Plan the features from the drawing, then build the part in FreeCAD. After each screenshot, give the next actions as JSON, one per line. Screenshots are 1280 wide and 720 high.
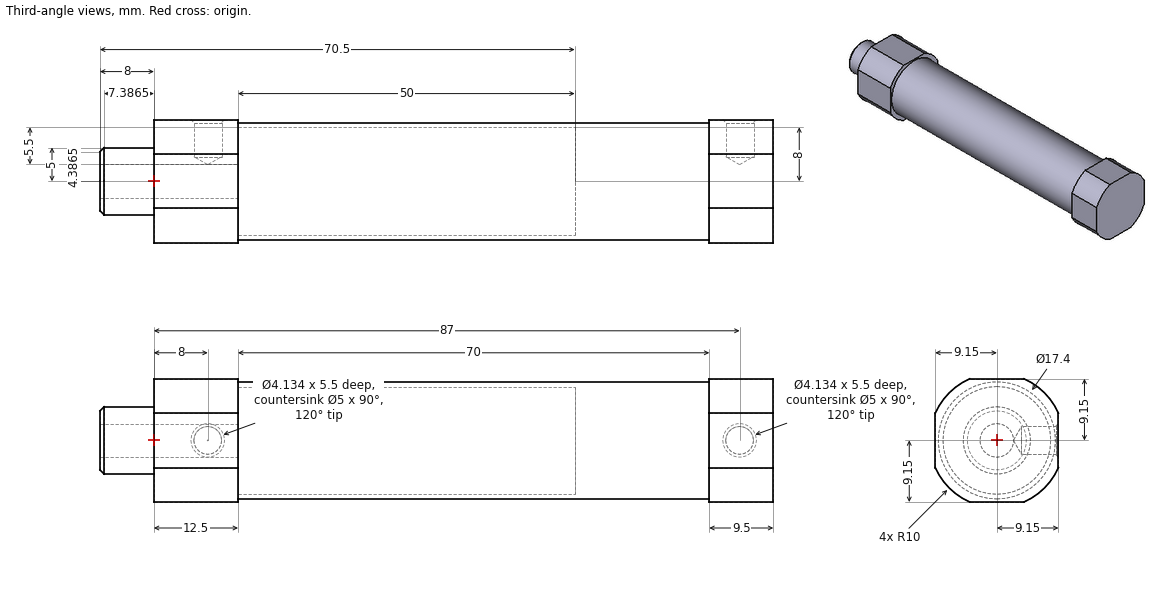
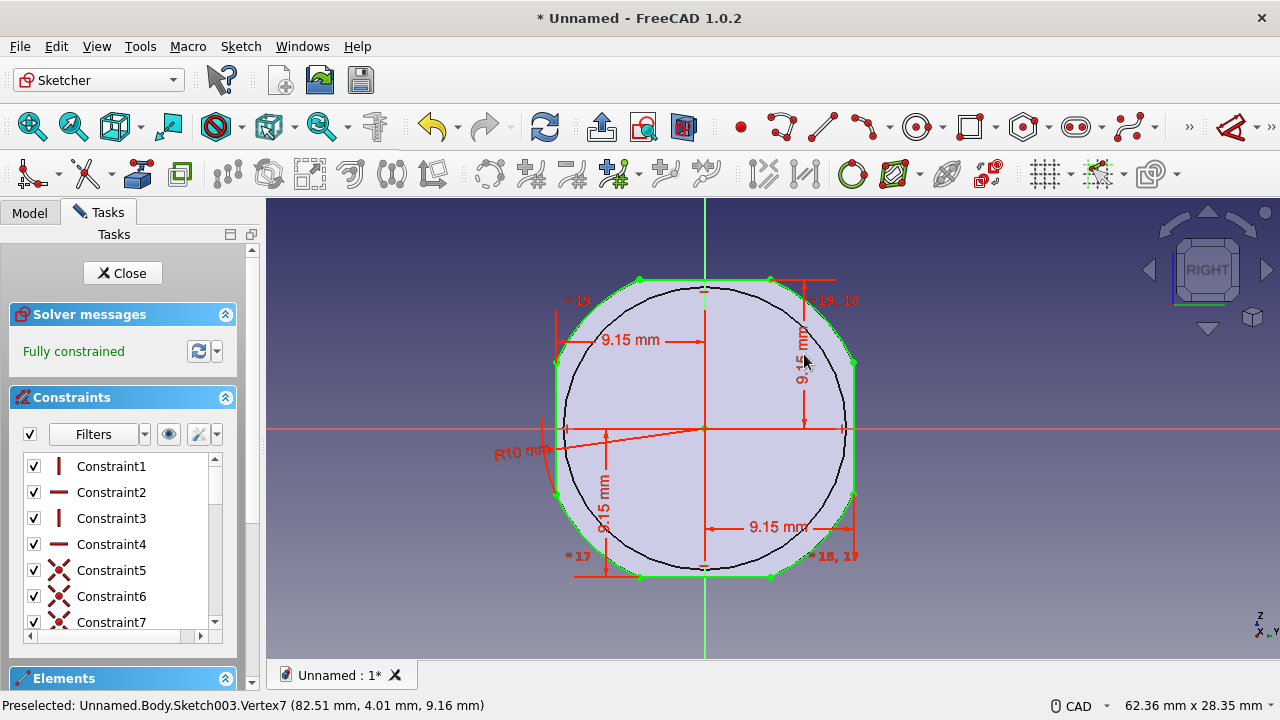
{"action": "left_click", "coordinate": [123, 273]}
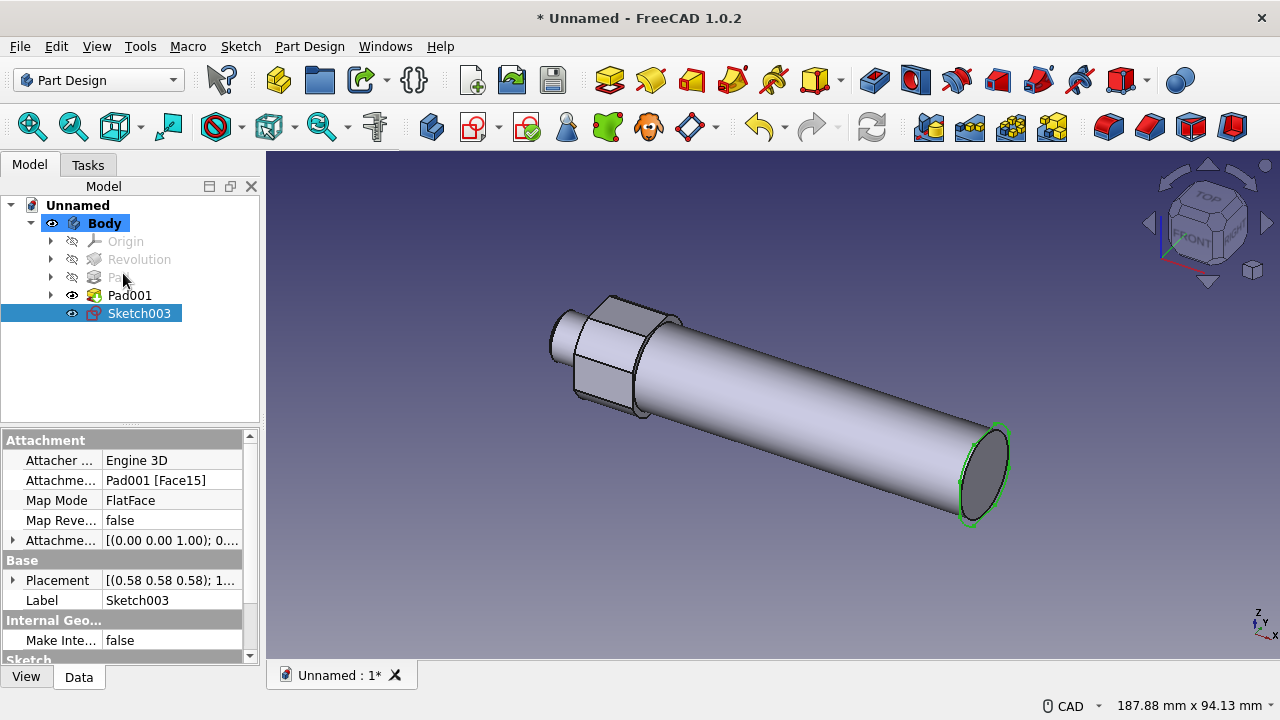
{"action": "left_click", "coordinate": [610, 80]}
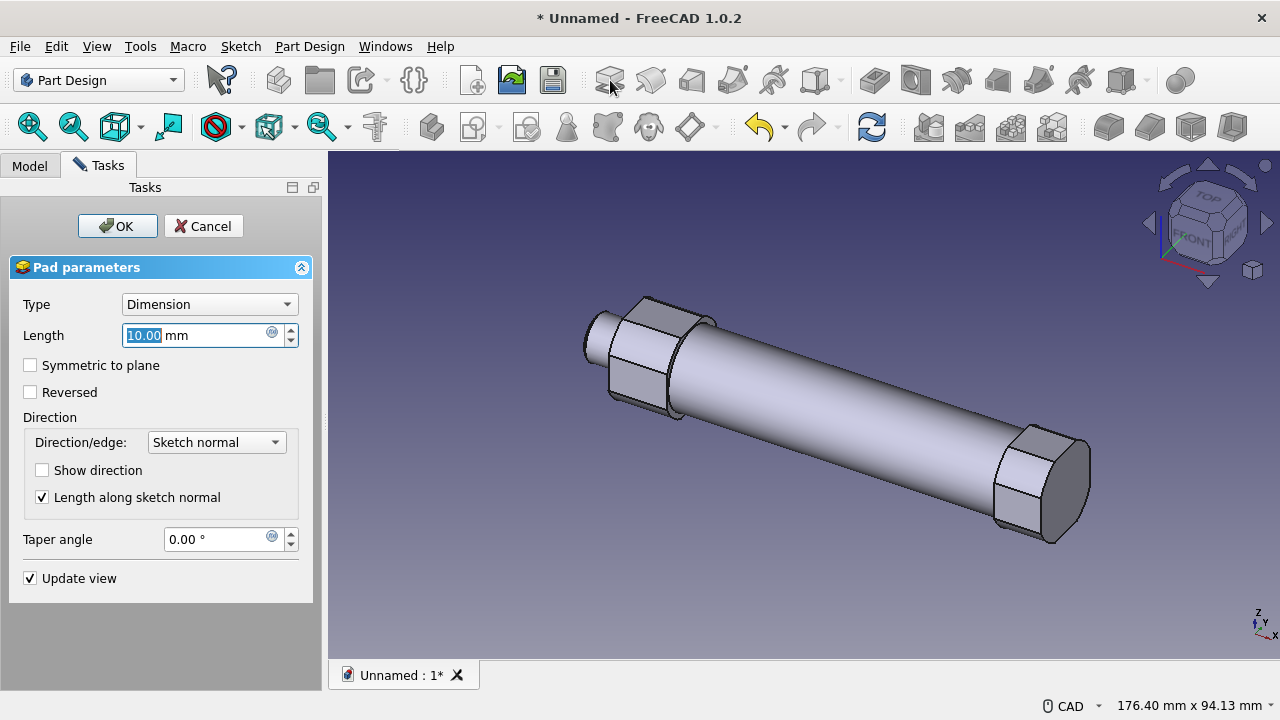
{"action": "type", "text": "9.5"}
{"action": "key", "text": "Tab"}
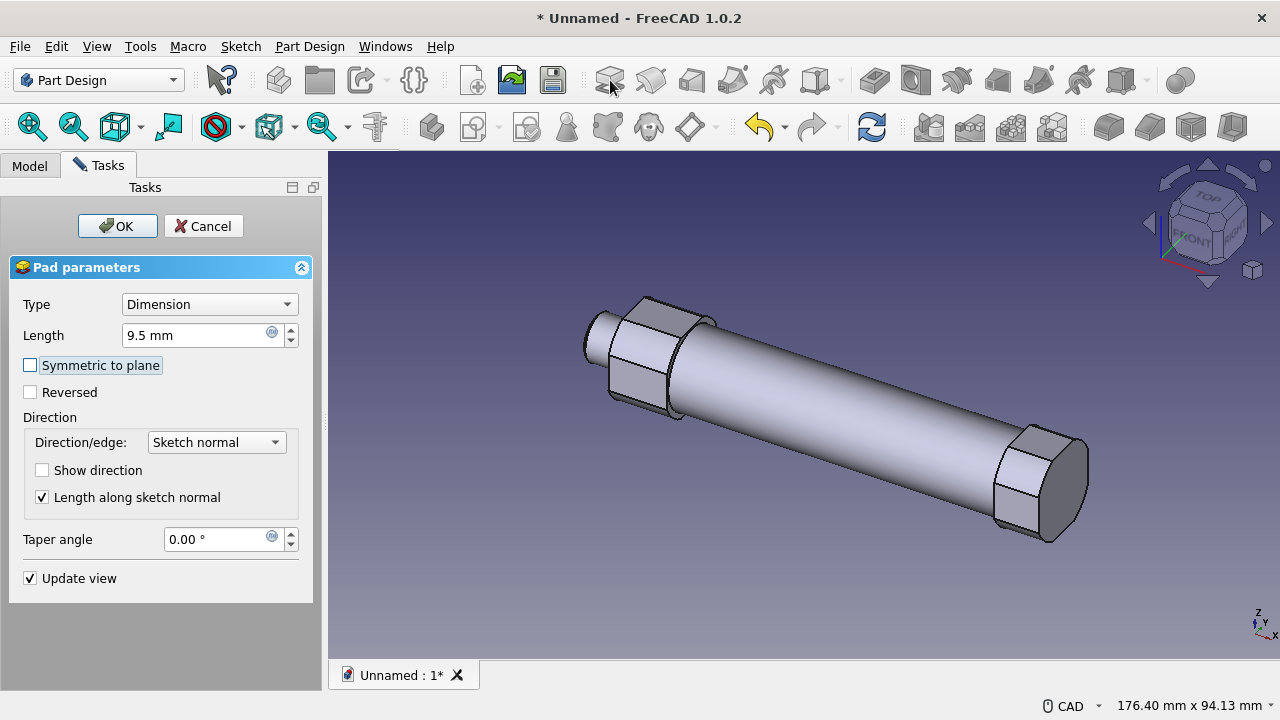
{"action": "left_click", "coordinate": [118, 226]}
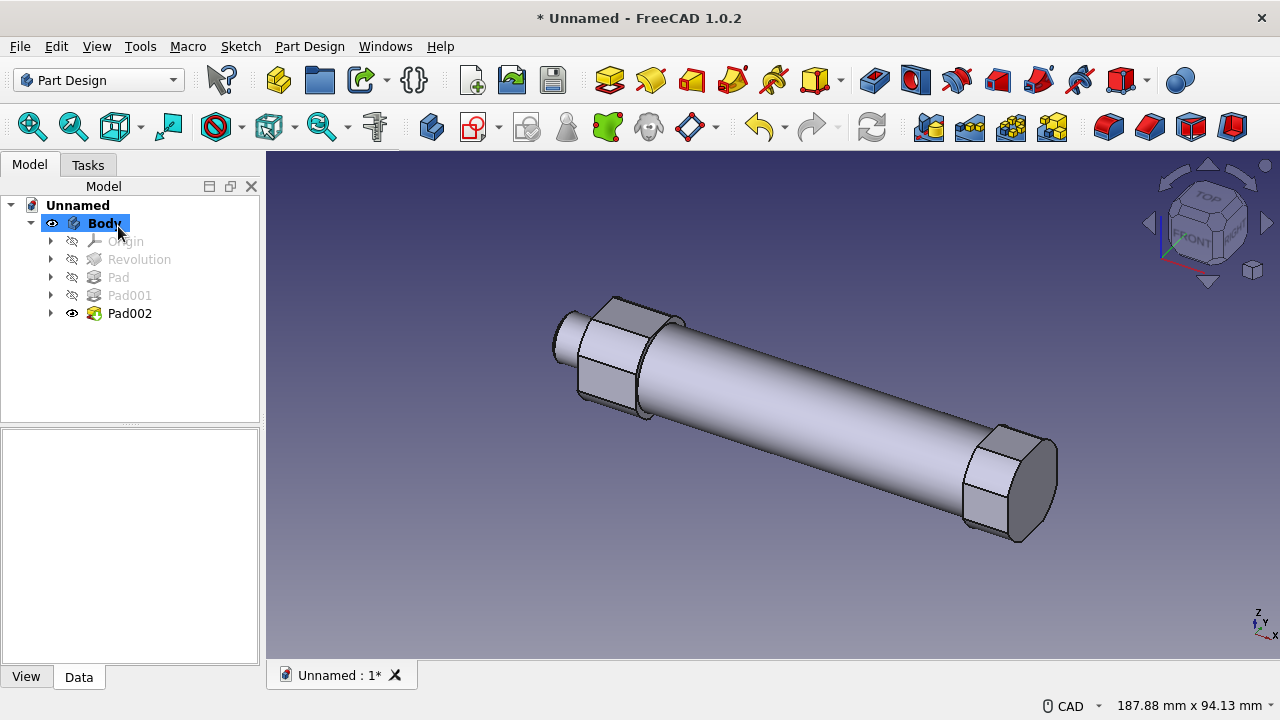
{"action": "key", "text": "4"}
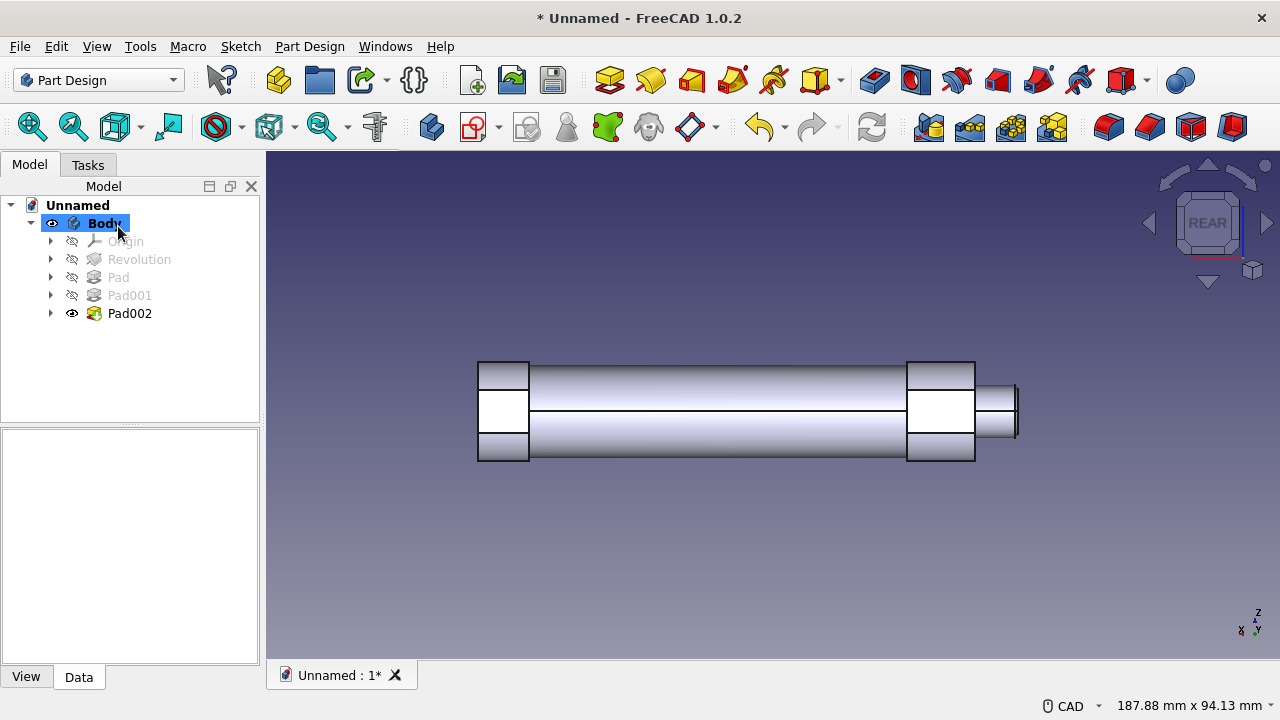
{"action": "left_click", "coordinate": [931, 410]}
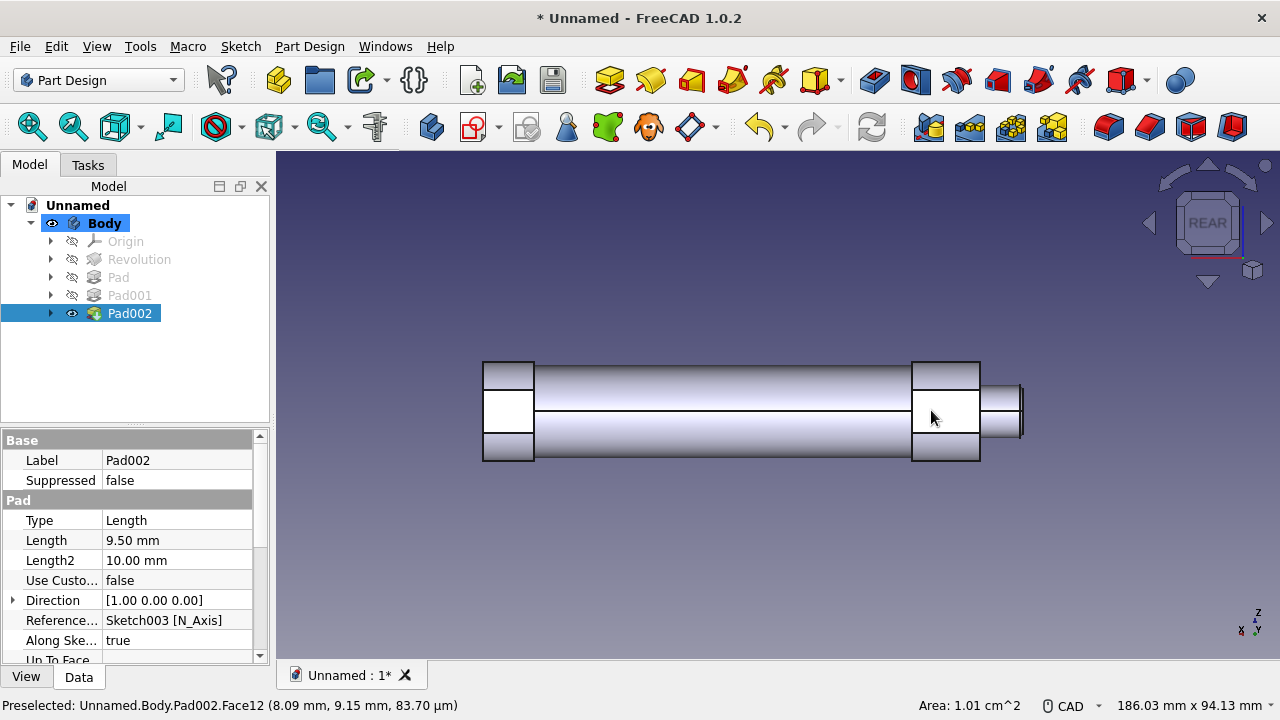
{"action": "left_click", "coordinate": [472, 128]}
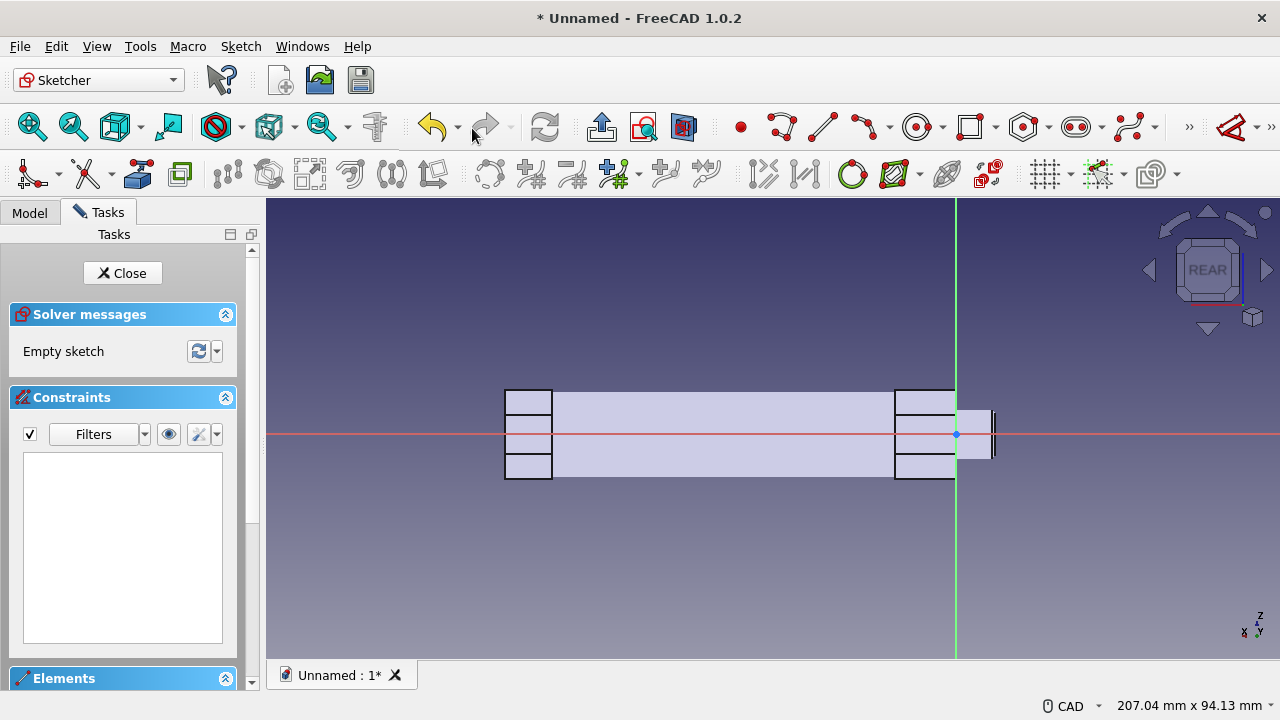
{"action": "scroll", "coordinate": [954, 435], "scroll_direction": "up", "scroll_amount": 12}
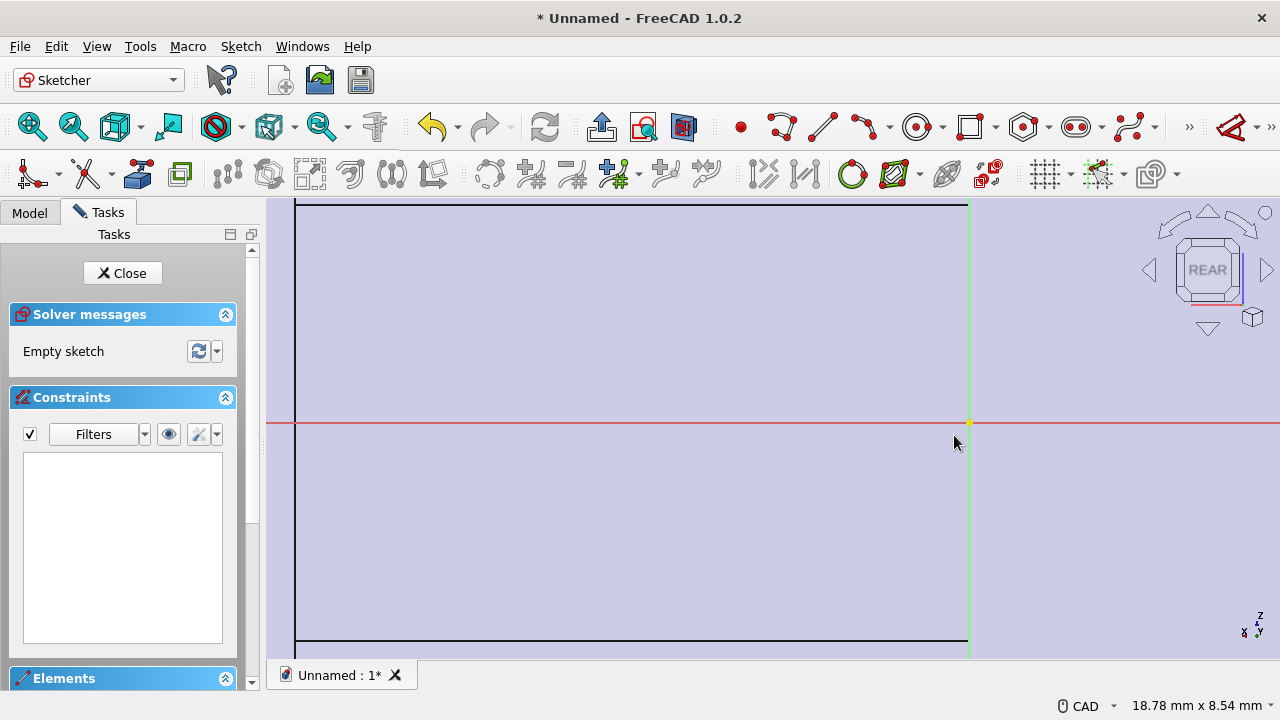
{"action": "left_click", "coordinate": [916, 128]}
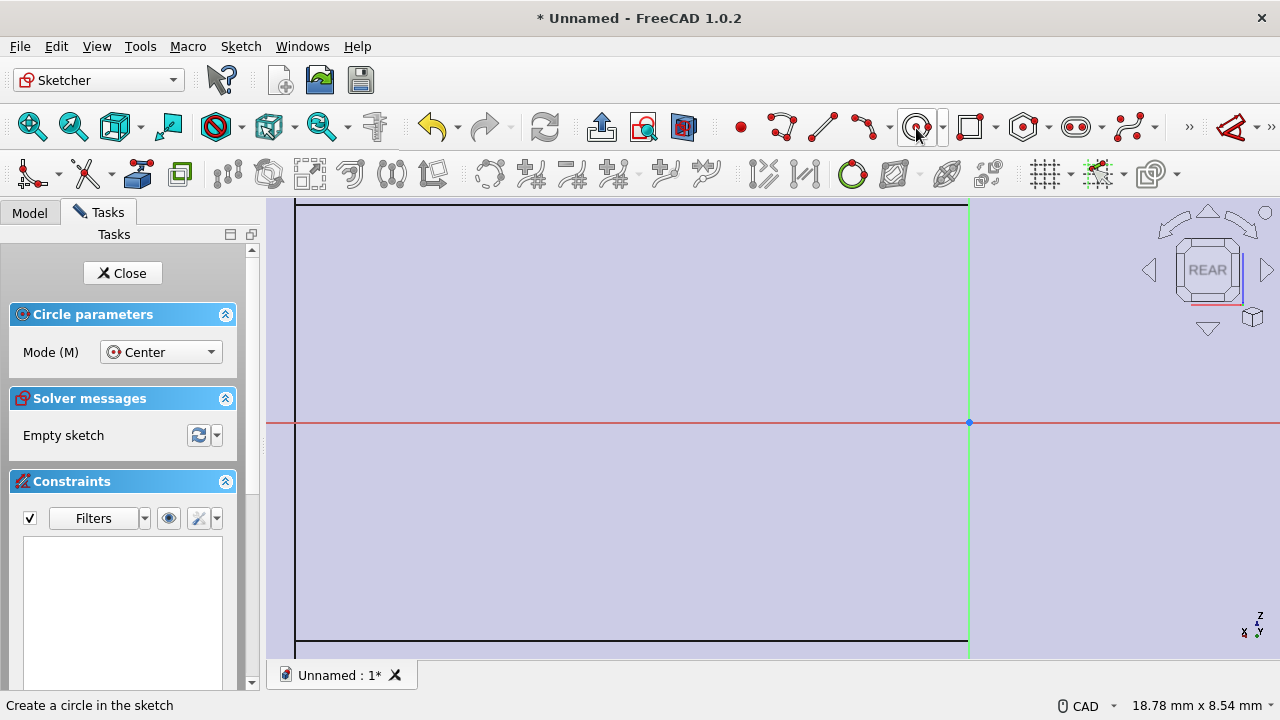
{"action": "left_click", "coordinate": [538, 423]}
{"action": "left_click", "coordinate": [616, 344]}
{"action": "key", "text": "Escape"}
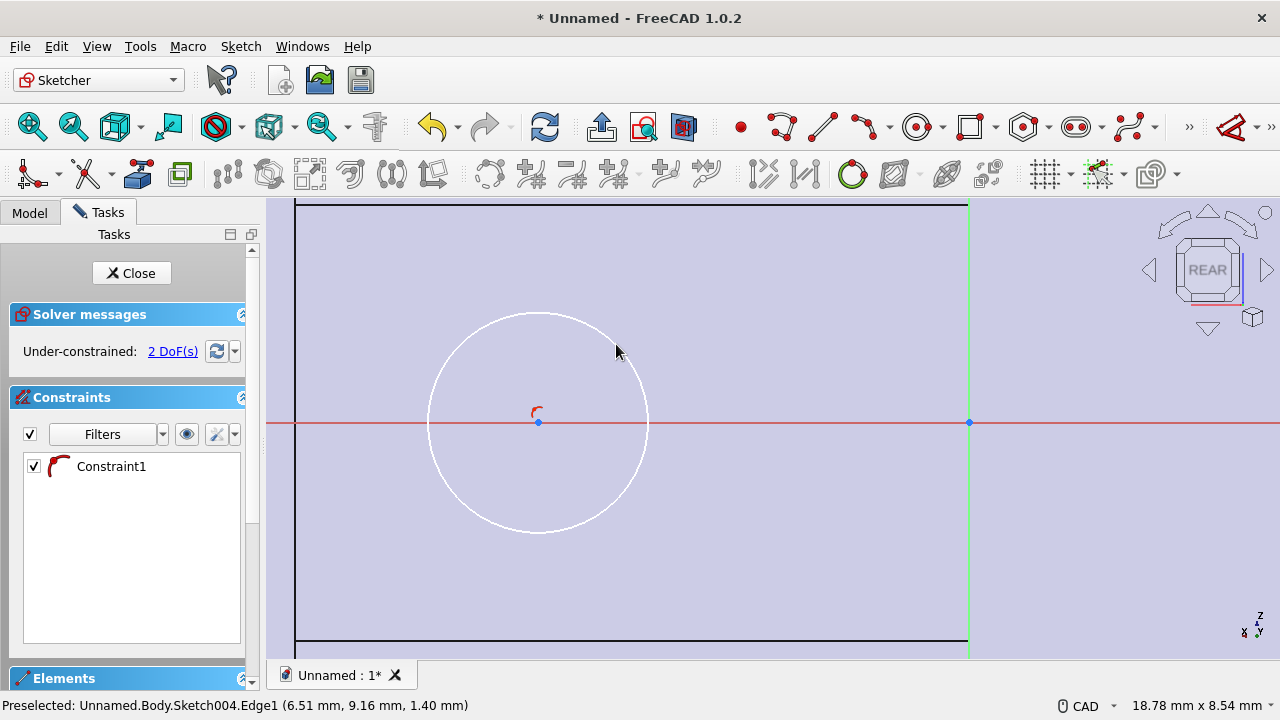
{"action": "left_click", "coordinate": [1230, 128]}